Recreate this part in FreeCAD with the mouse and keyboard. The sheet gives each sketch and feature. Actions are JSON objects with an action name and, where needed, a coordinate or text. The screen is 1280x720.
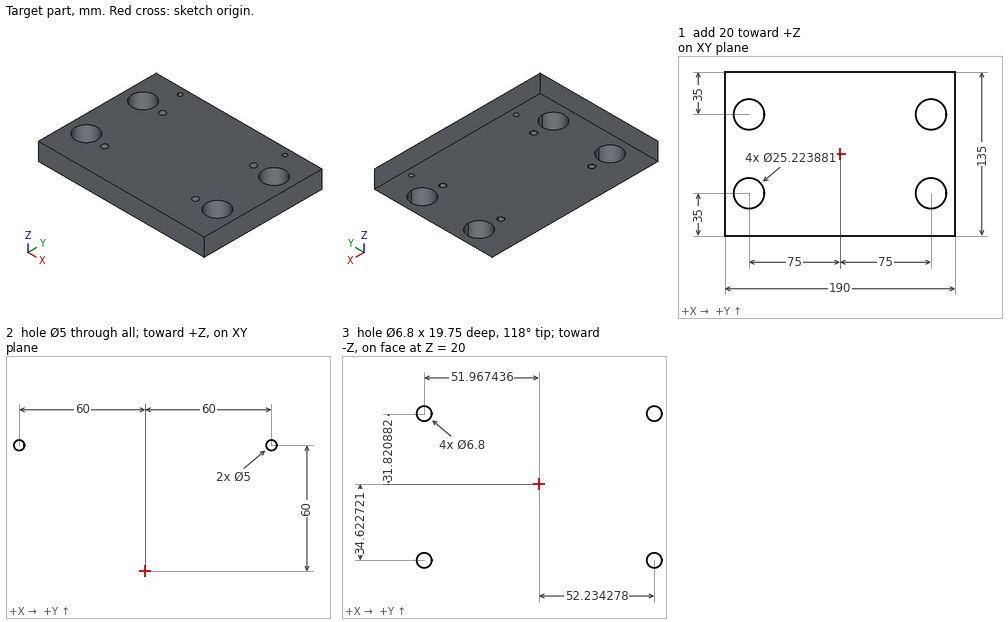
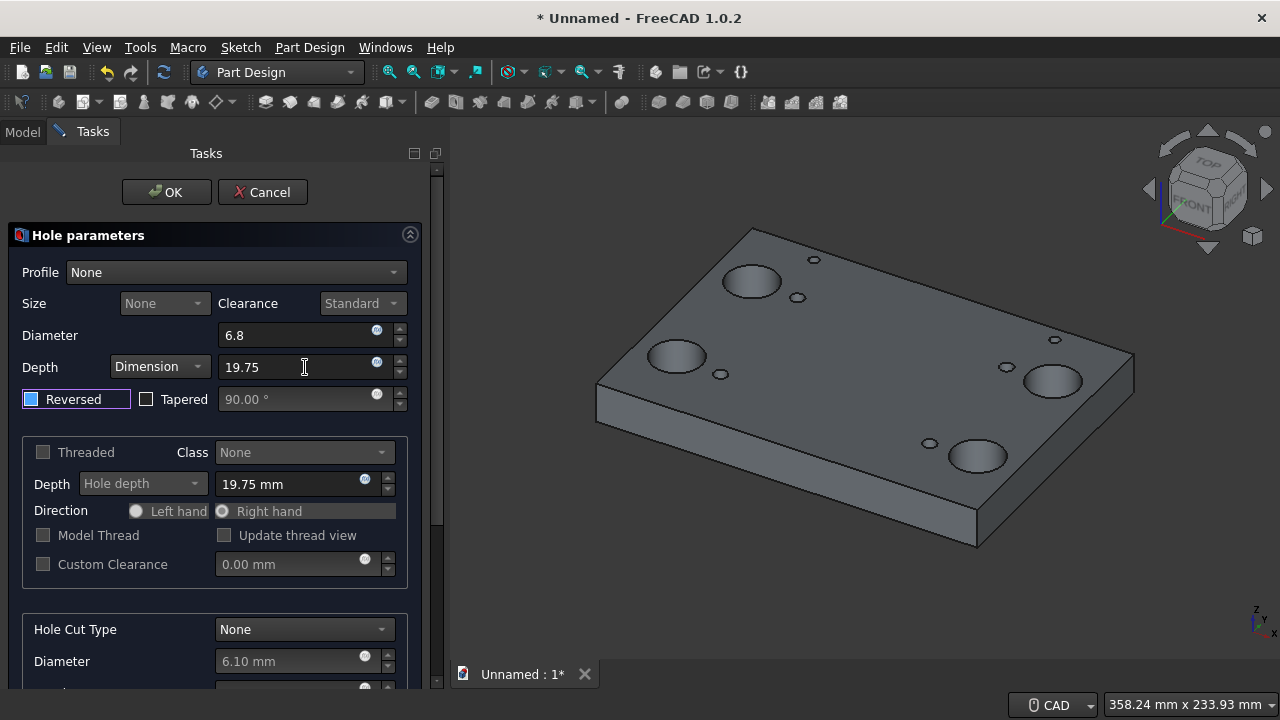
{"action": "left_click", "coordinate": [167, 192]}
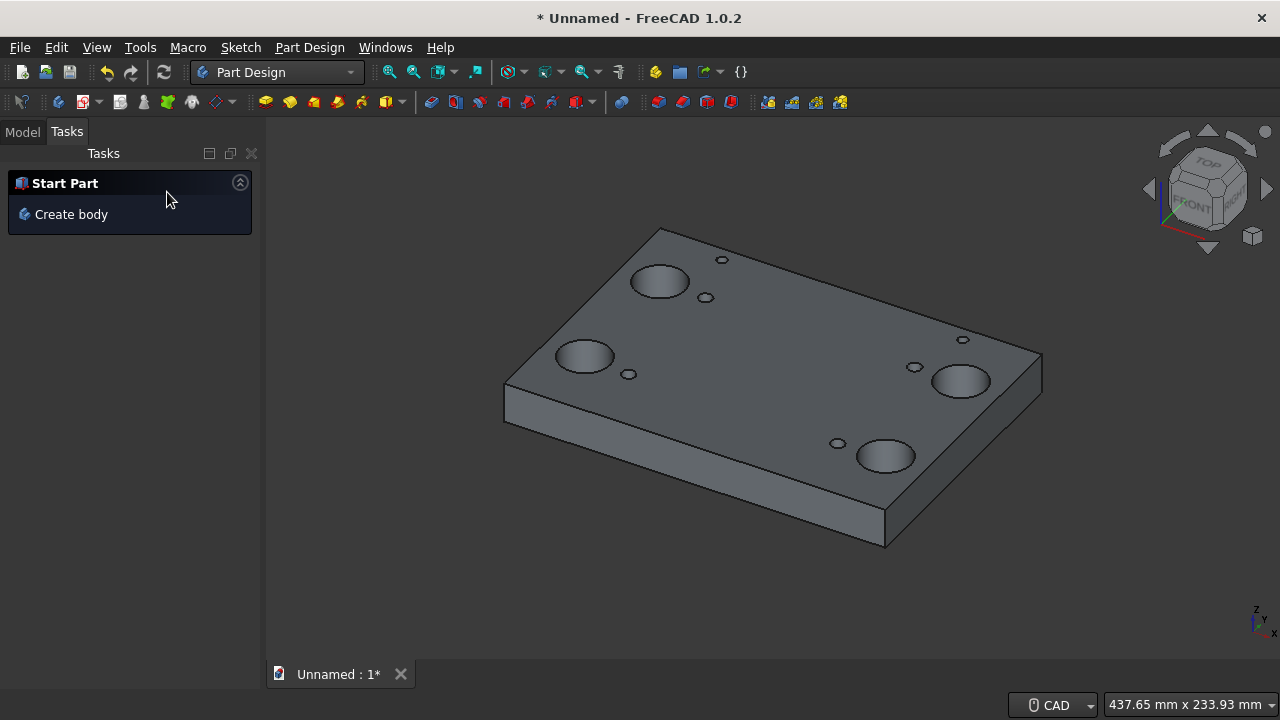
{"action": "key", "text": "0"}